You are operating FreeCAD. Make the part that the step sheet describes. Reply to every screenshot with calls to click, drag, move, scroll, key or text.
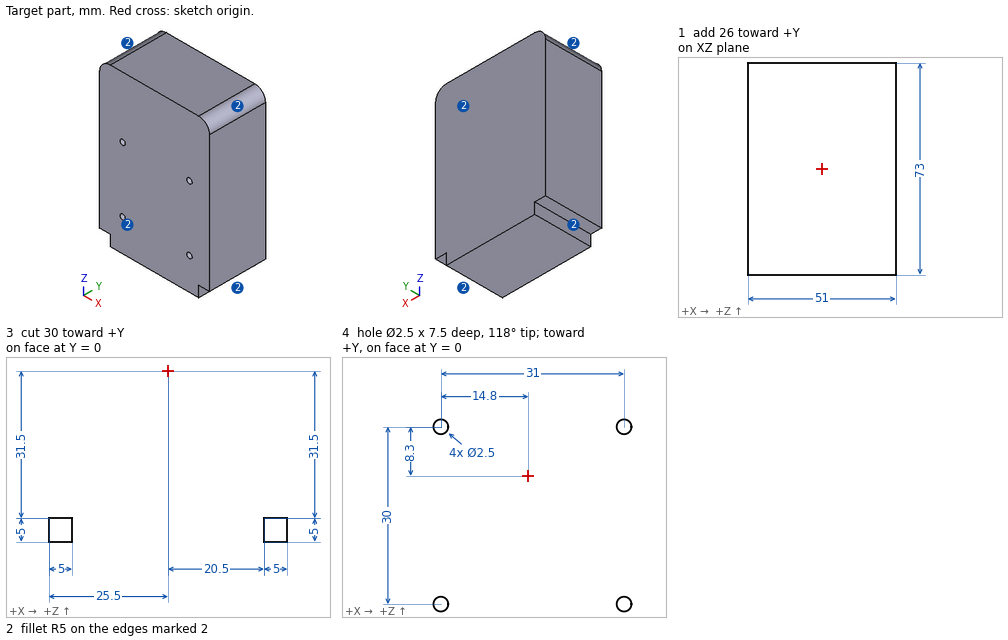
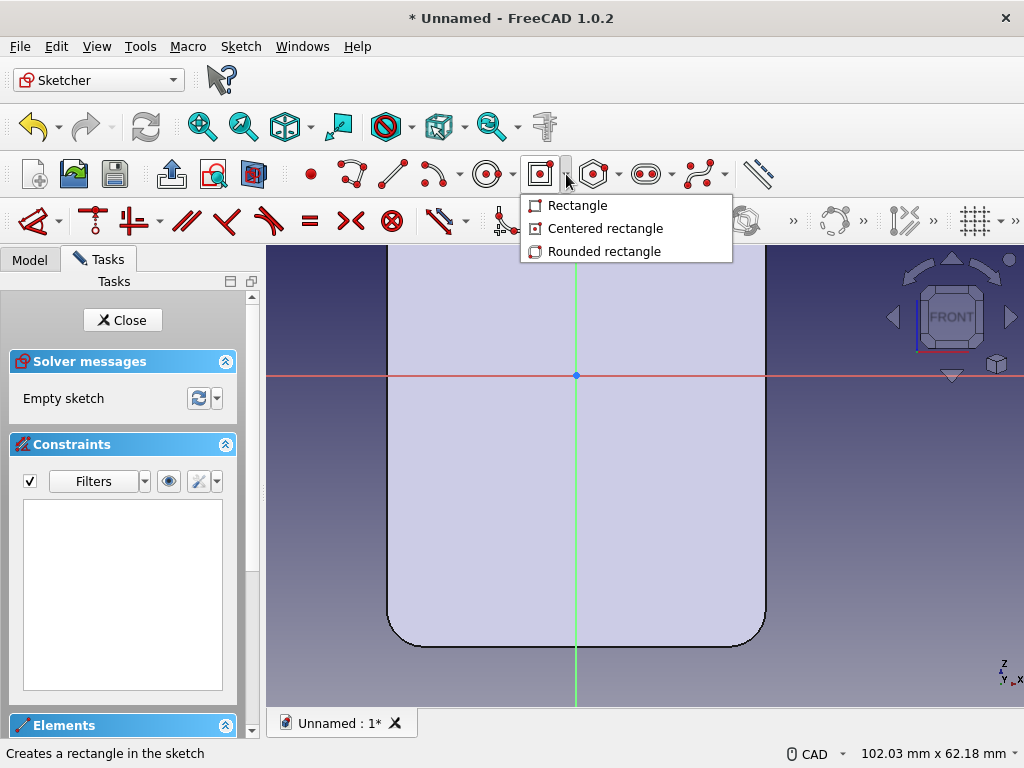
click(626, 206)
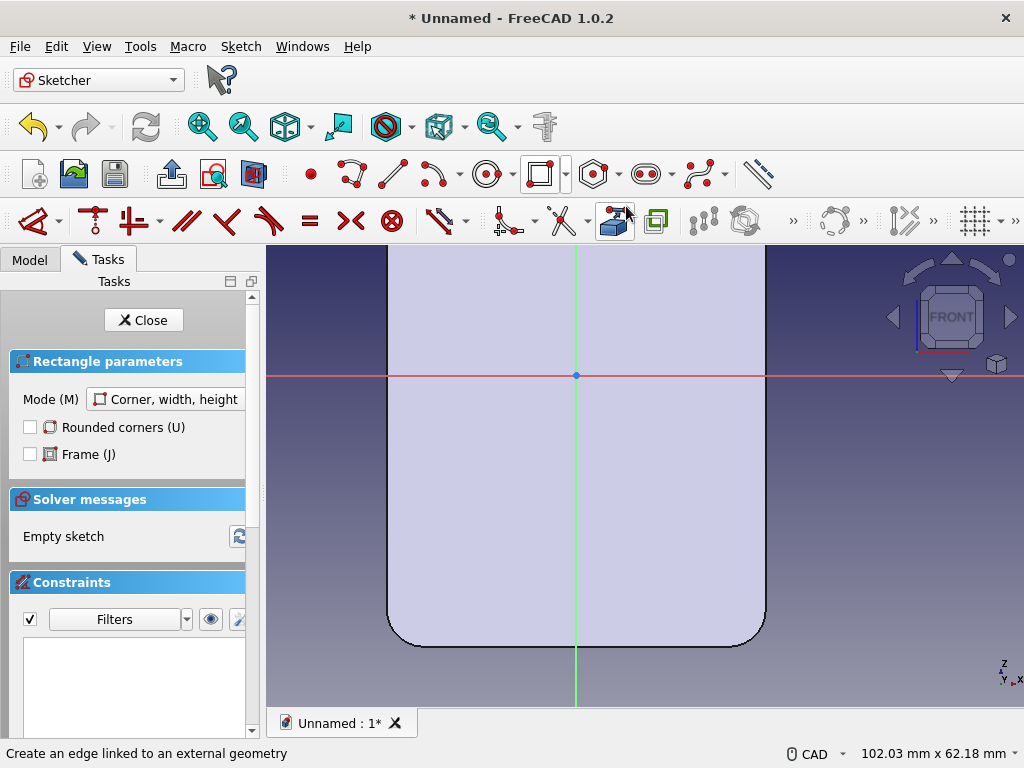
click(729, 610)
click(766, 647)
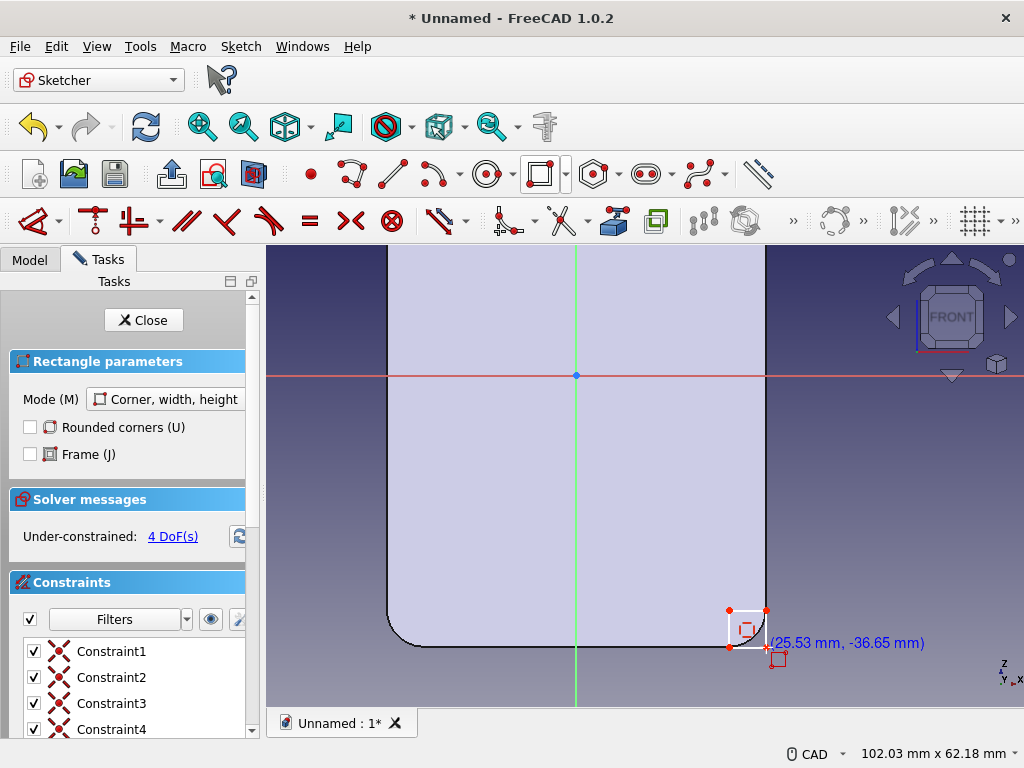
click(387, 610)
click(424, 647)
key(Escape)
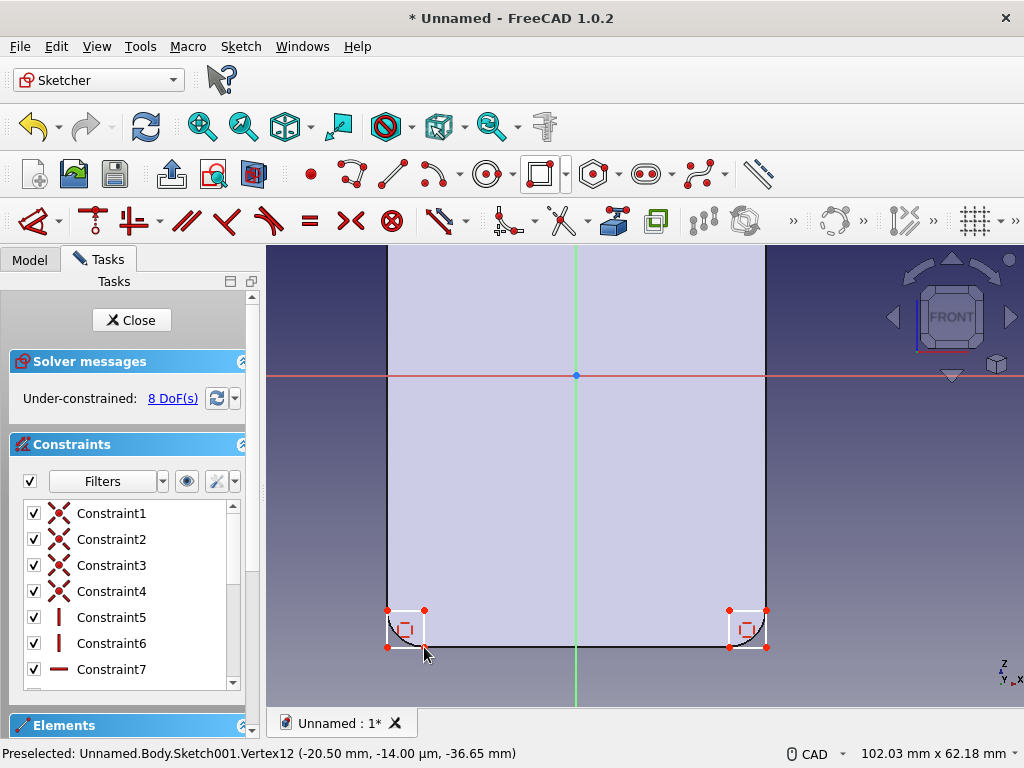
scroll(729, 622, up, 2)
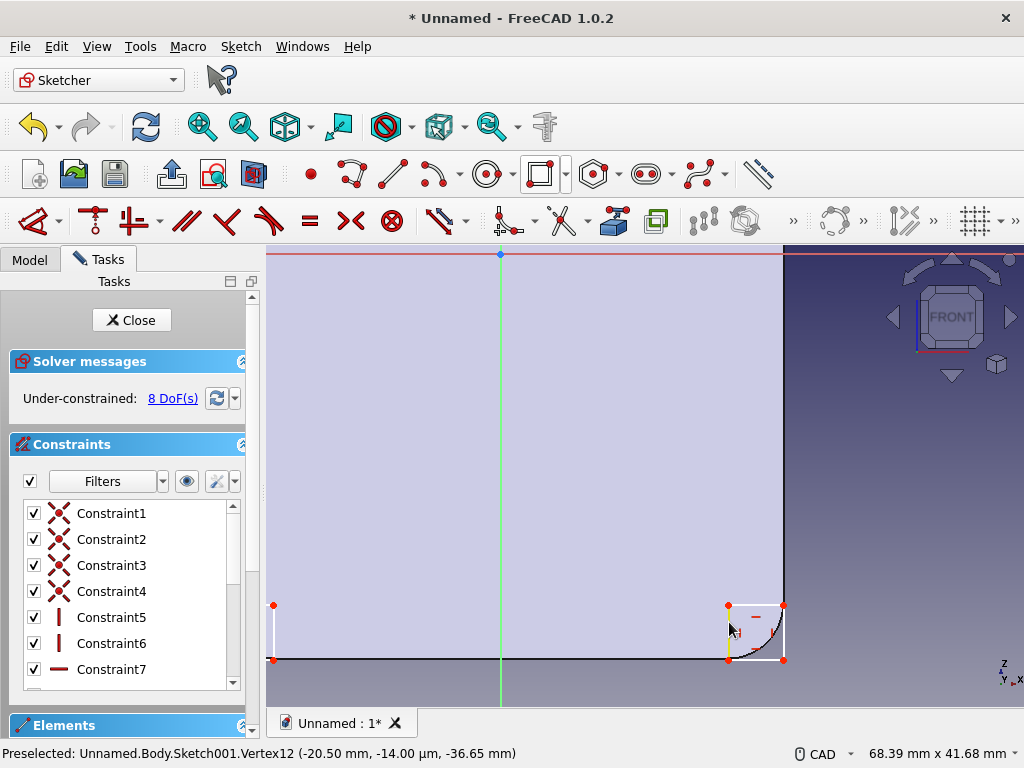
click(729, 622)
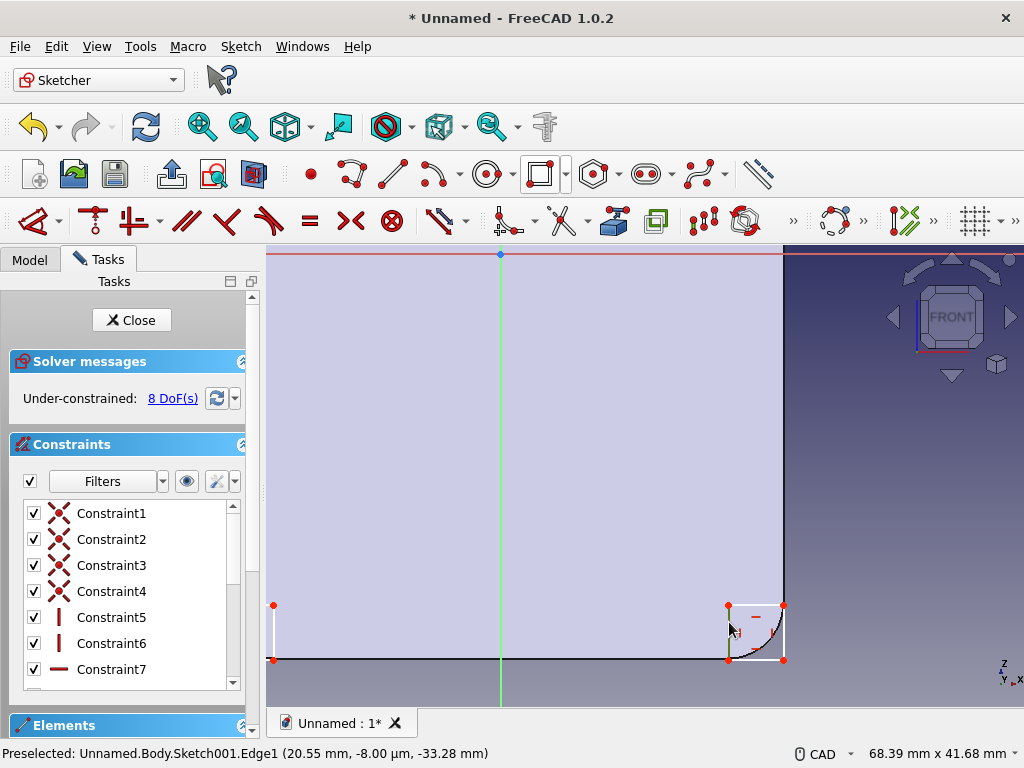
key(i)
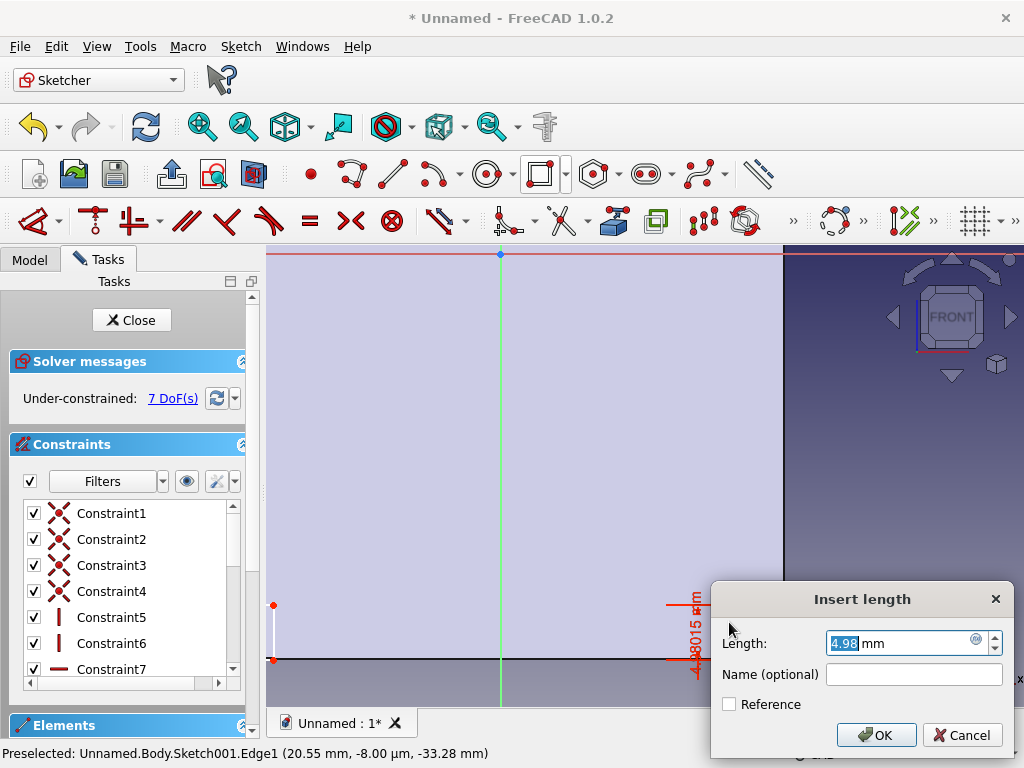
text(5)
key(Return)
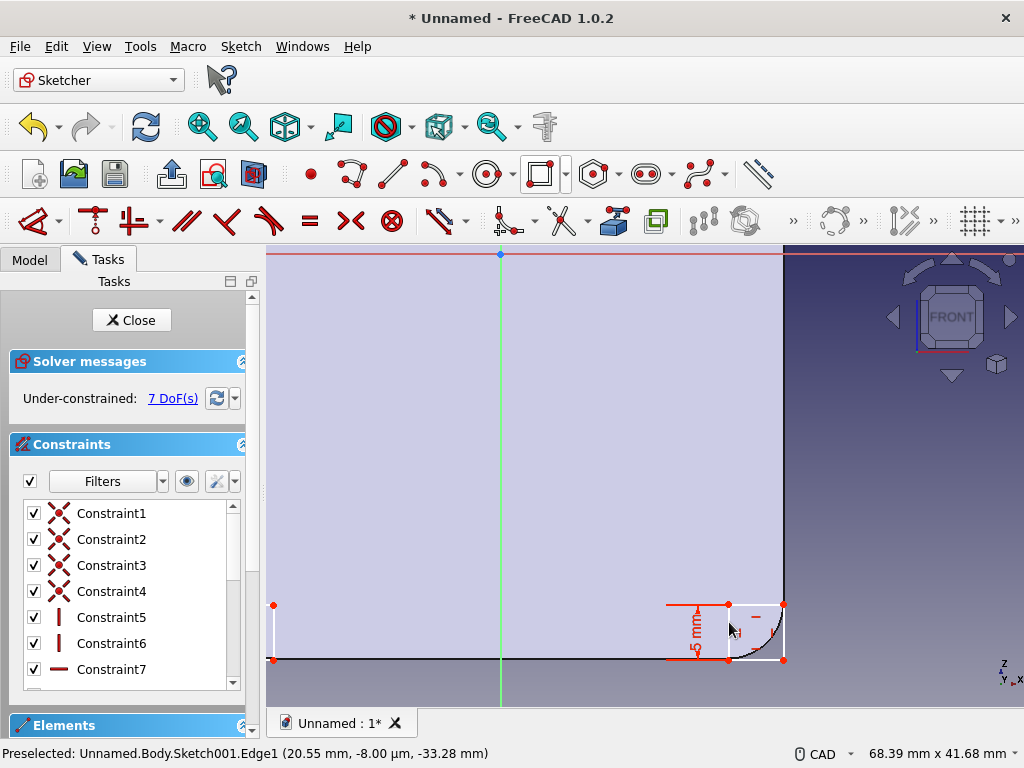
click(745, 660)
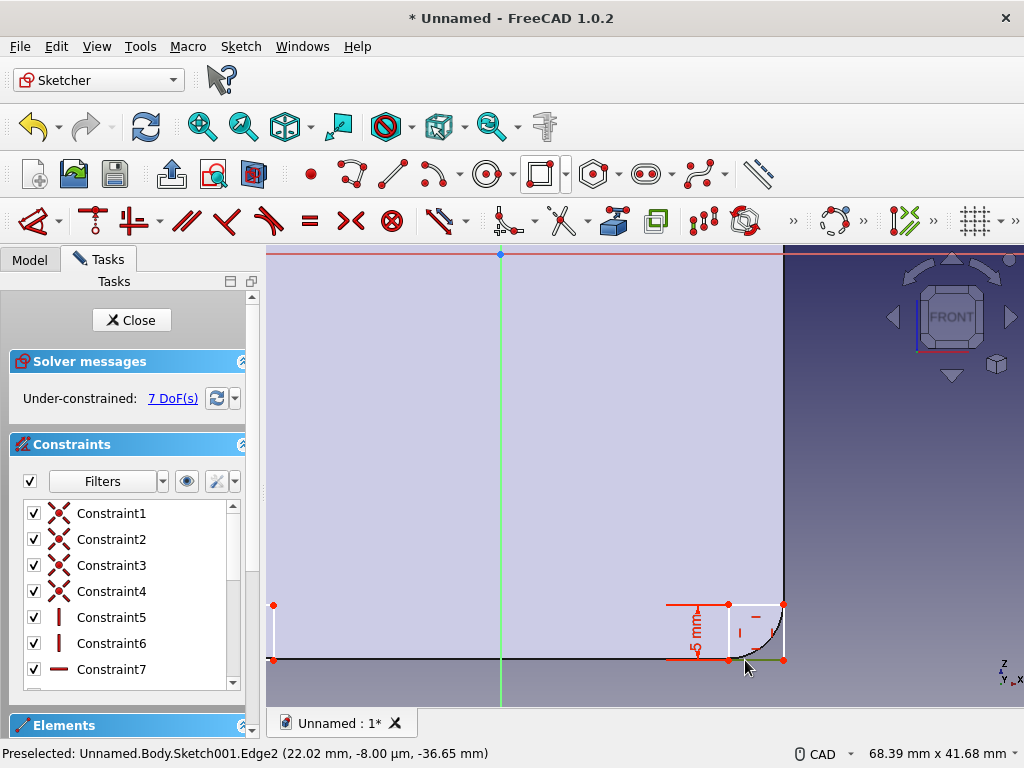
click(58, 222)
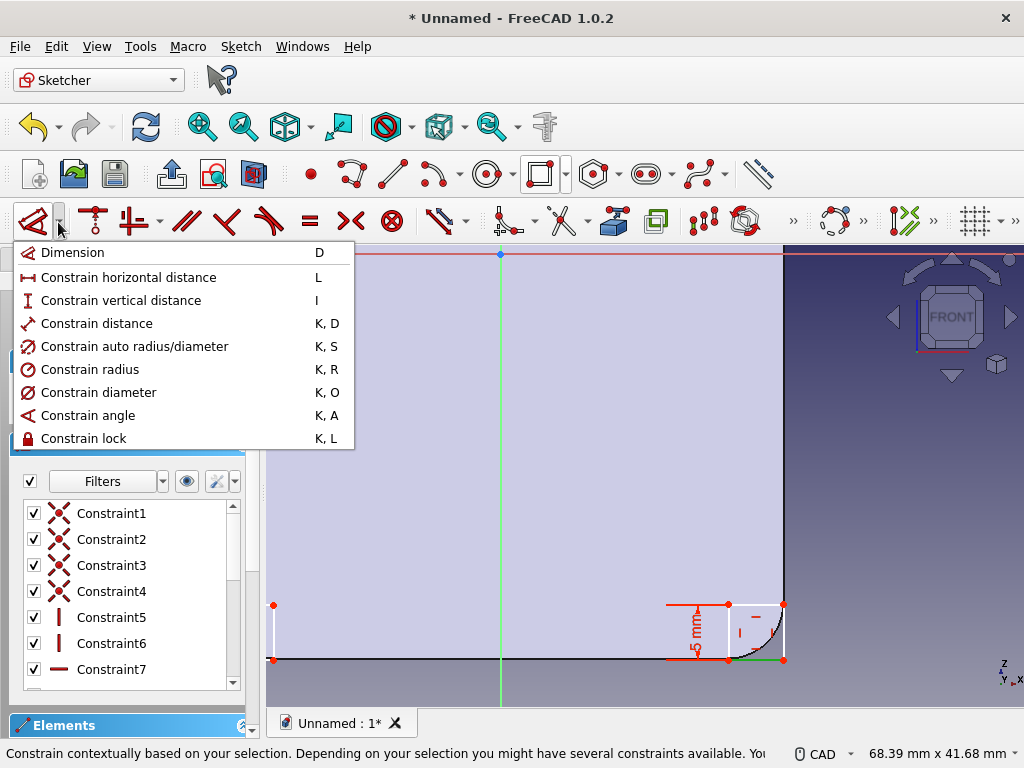
click(184, 278)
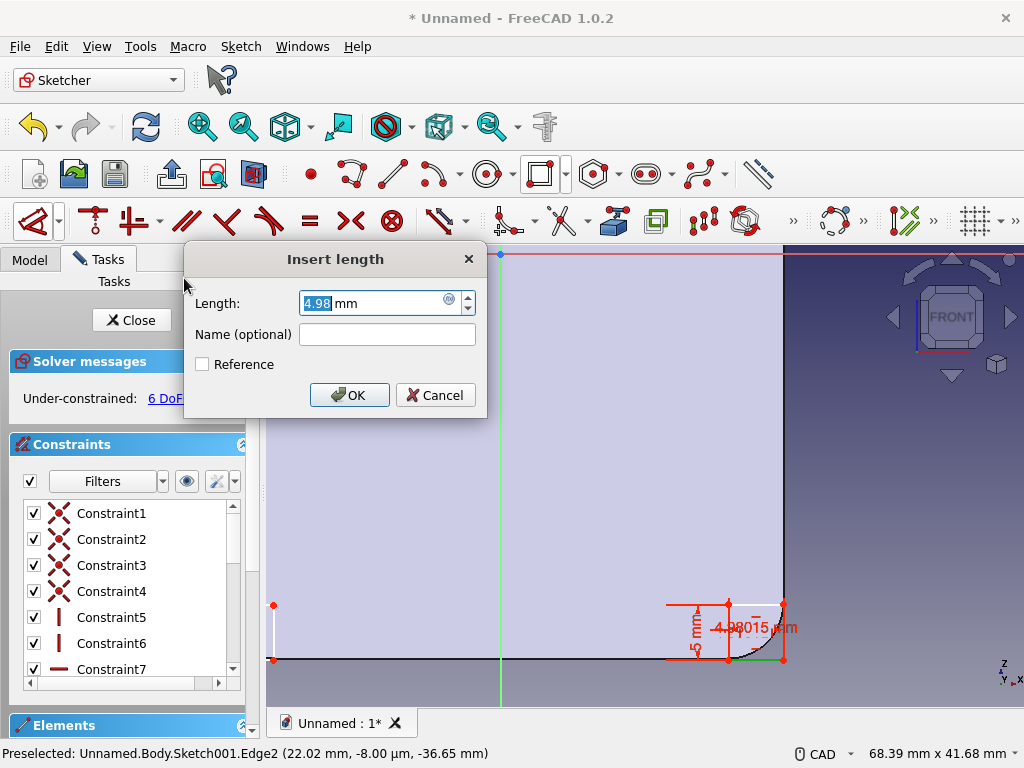
text(5)
key(Return)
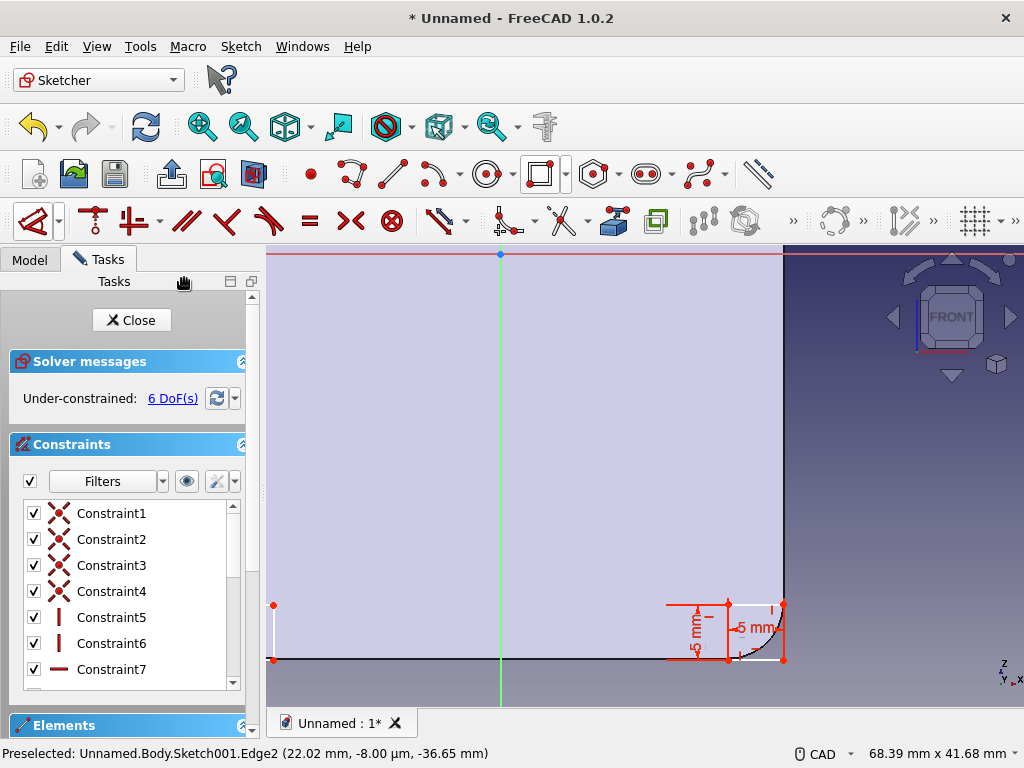
scroll(730, 516, down, 2)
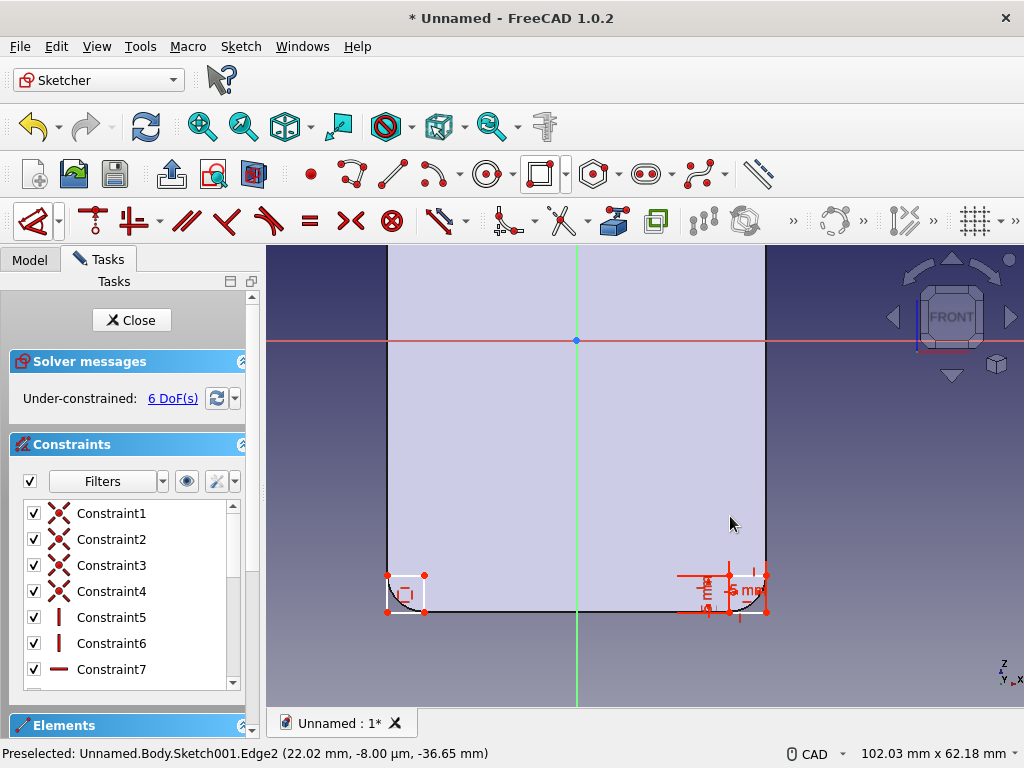
scroll(387, 587, up, 2)